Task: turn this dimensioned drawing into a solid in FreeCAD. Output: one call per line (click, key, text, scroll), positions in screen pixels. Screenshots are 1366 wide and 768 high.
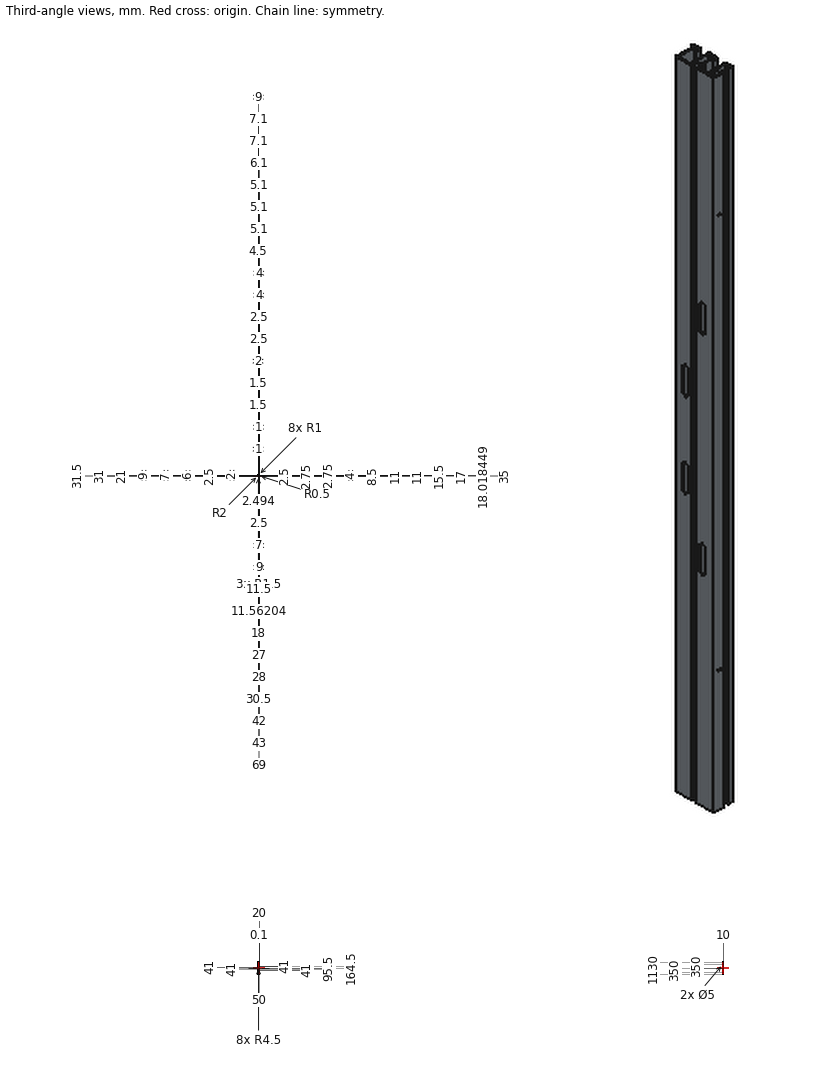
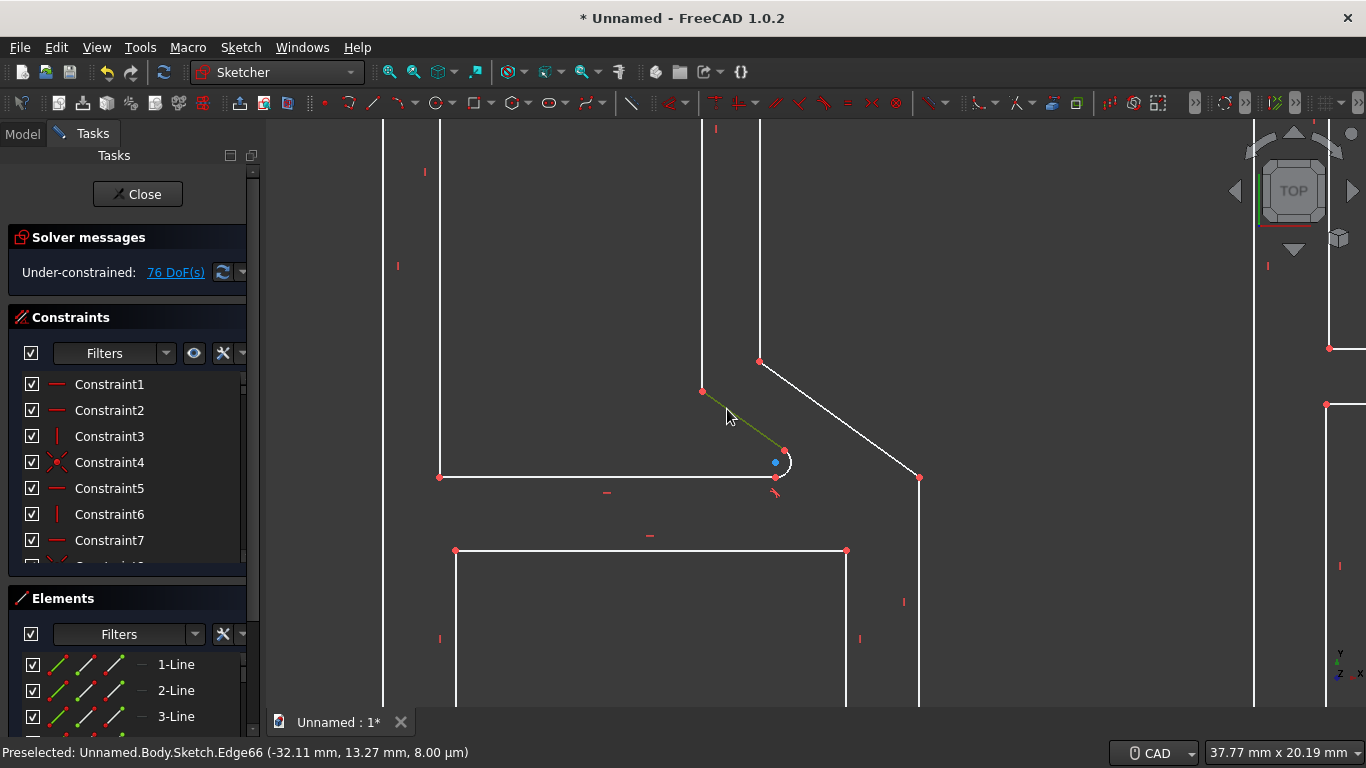
scroll(786, 473, up, 2)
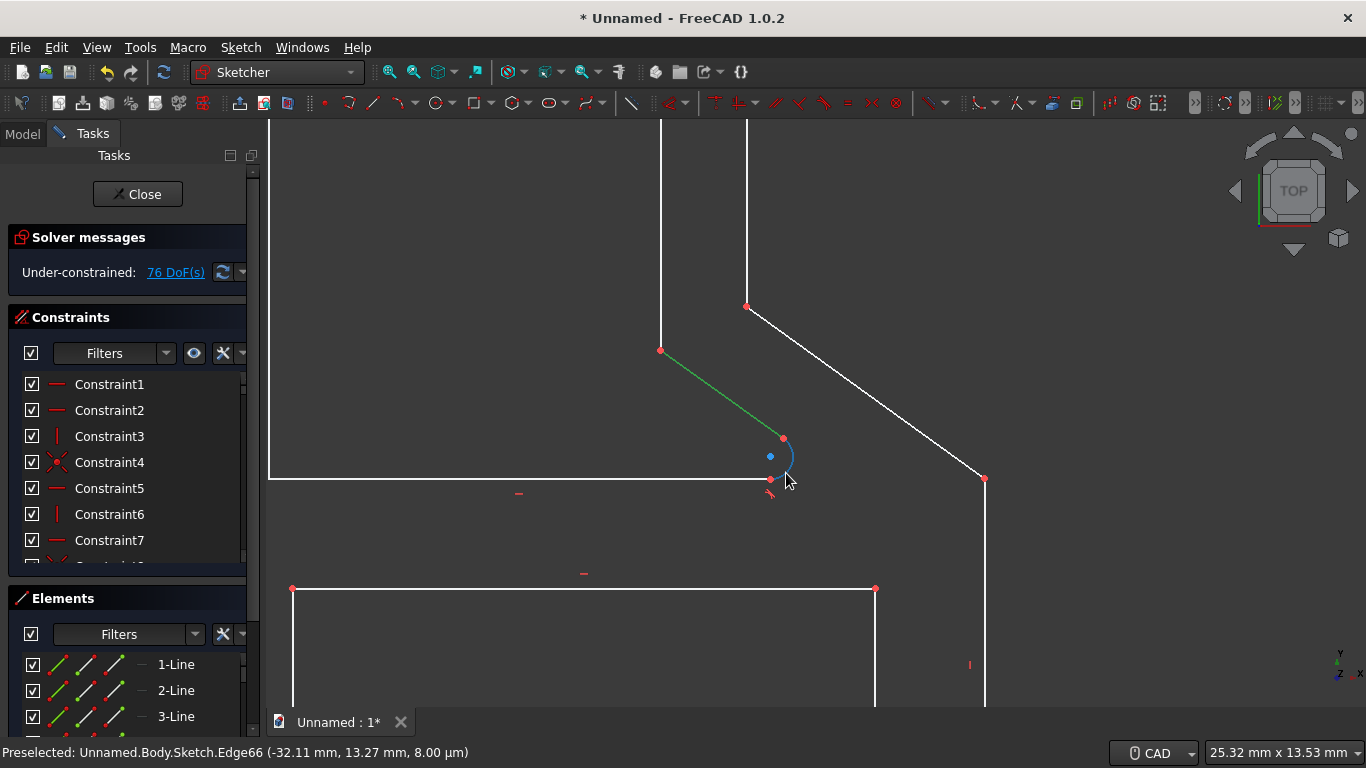
click(786, 473)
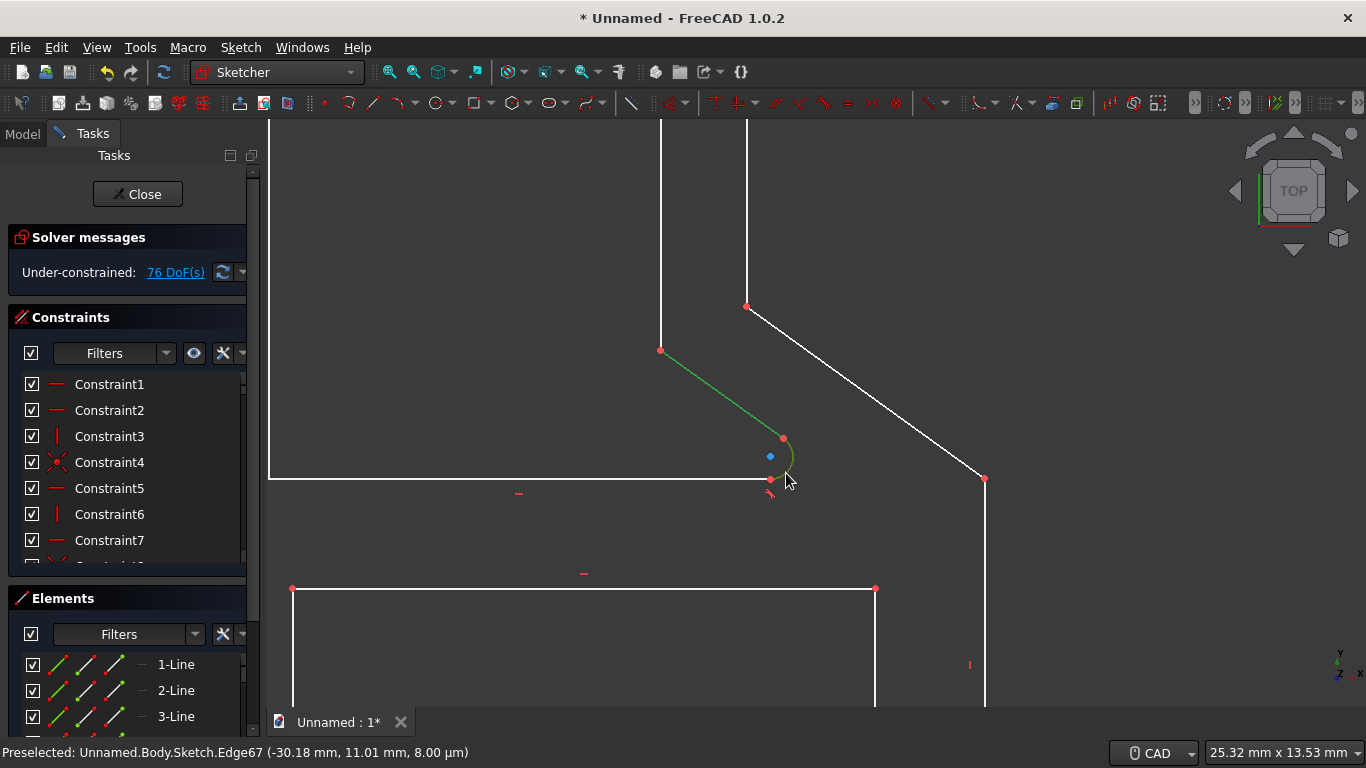
key(t)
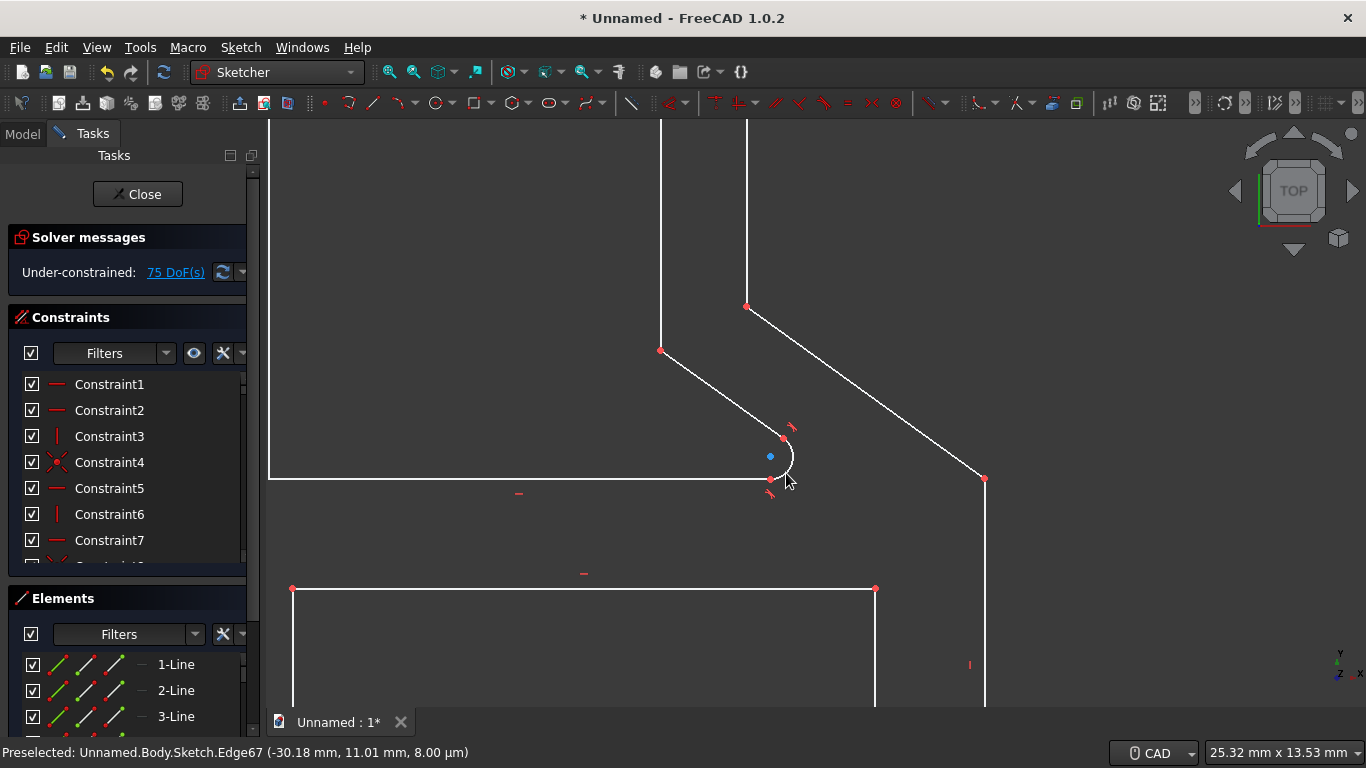
scroll(792, 468, down, 8)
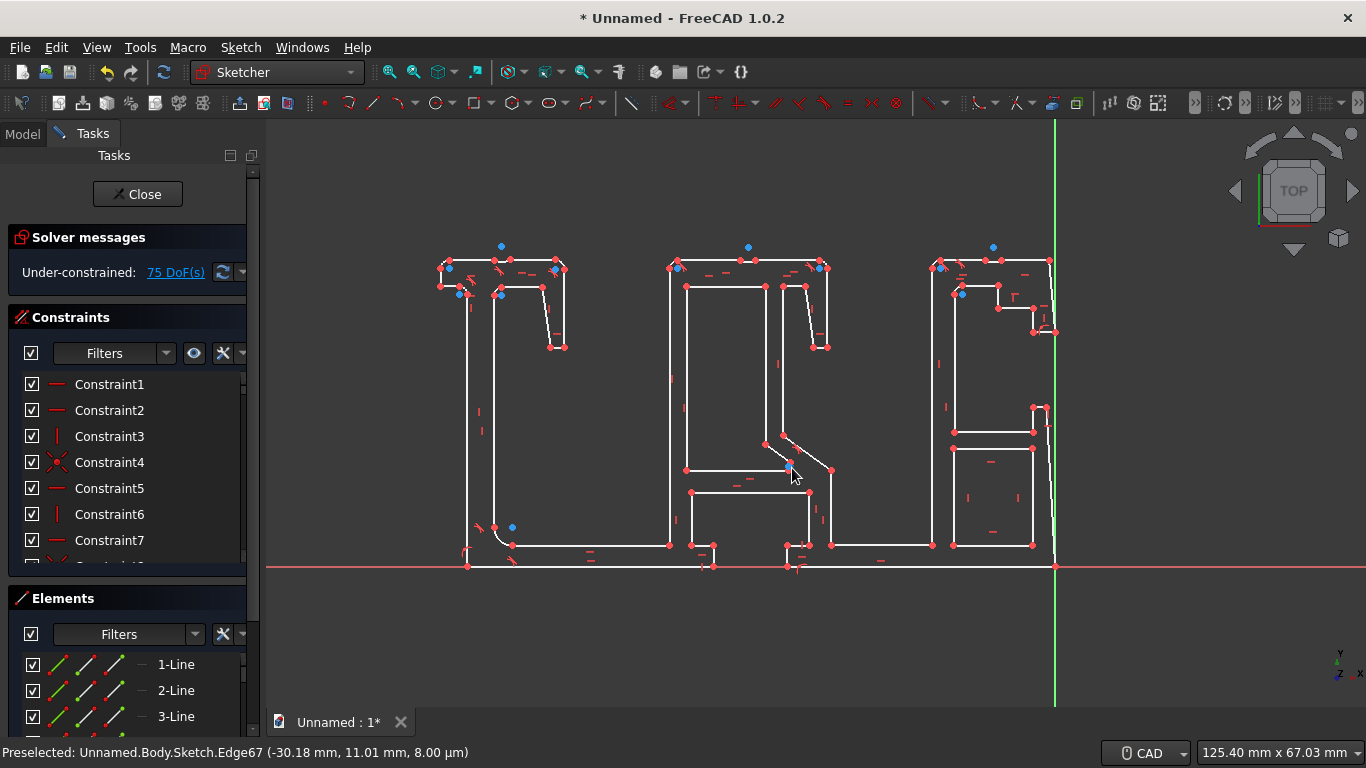
scroll(1053, 519, up, 9)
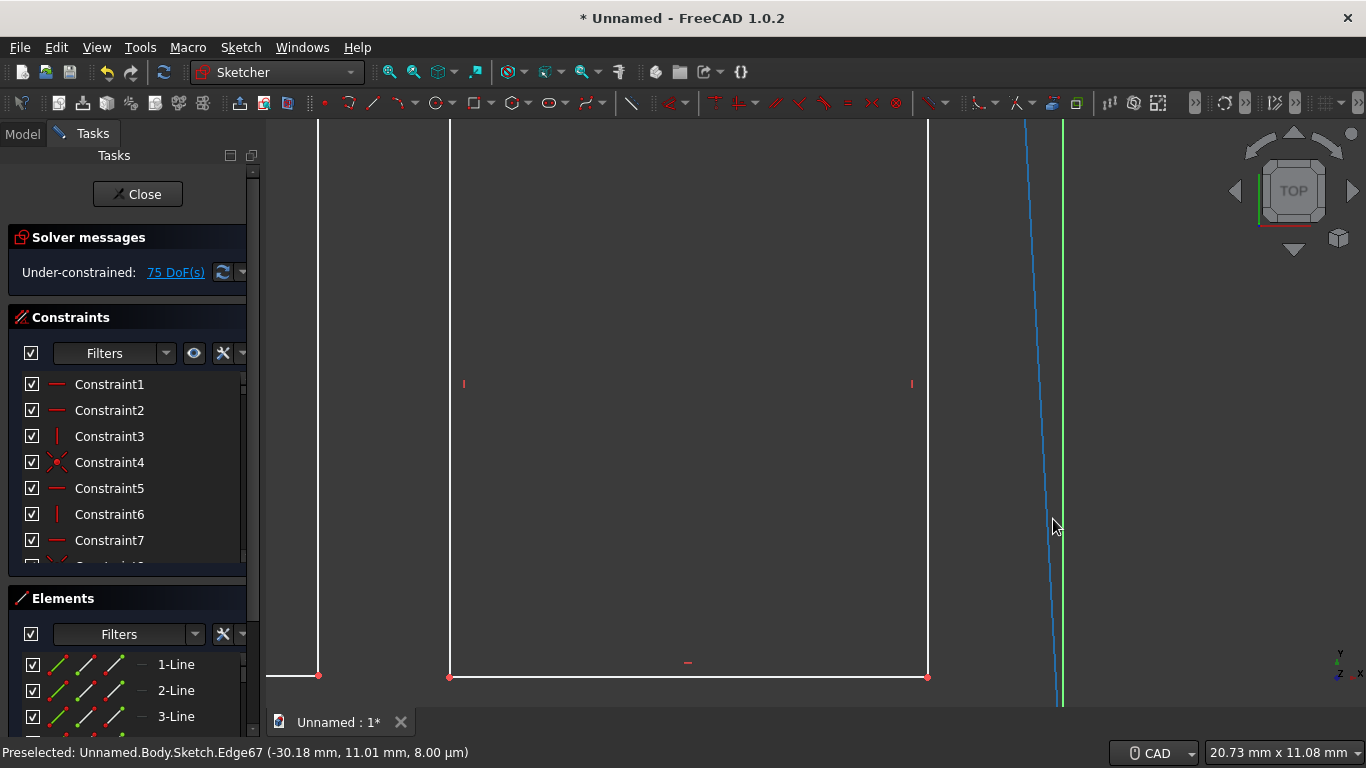
click(1047, 514)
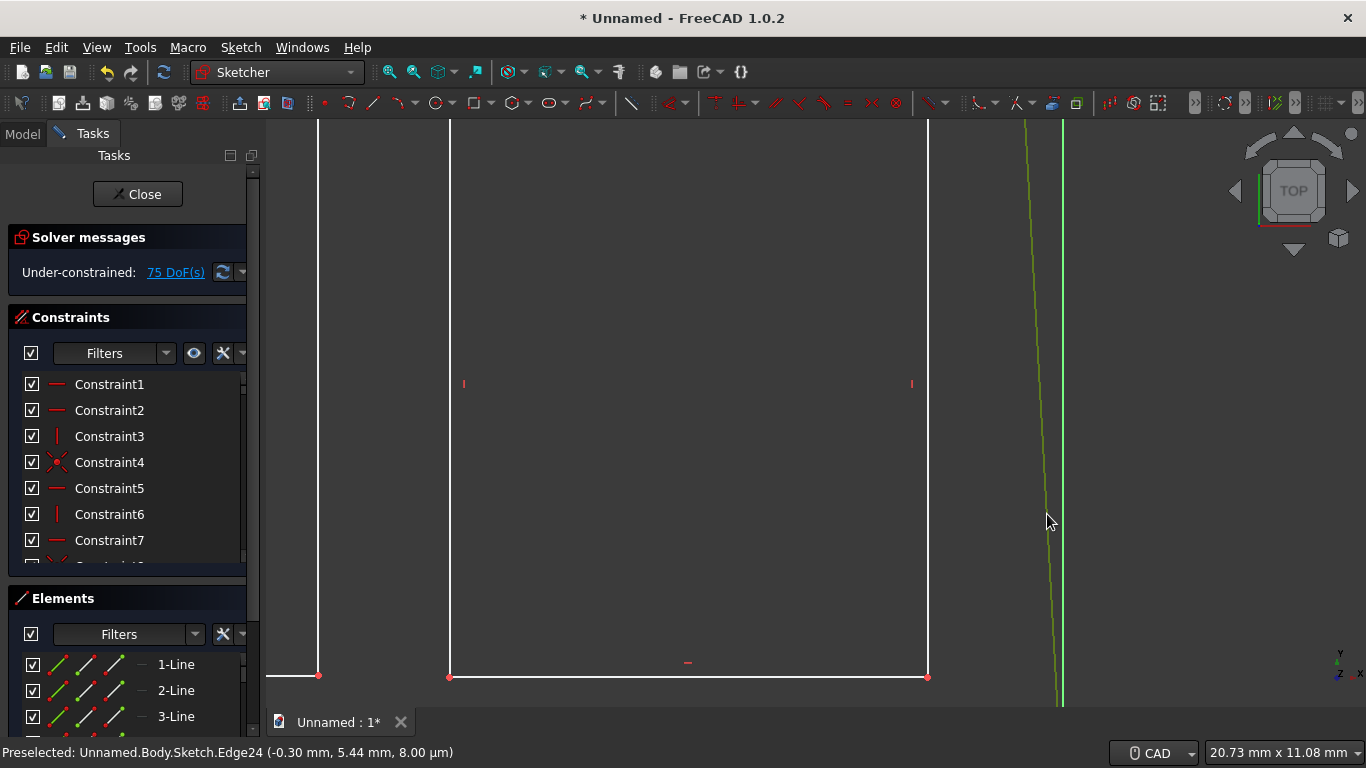
key(v)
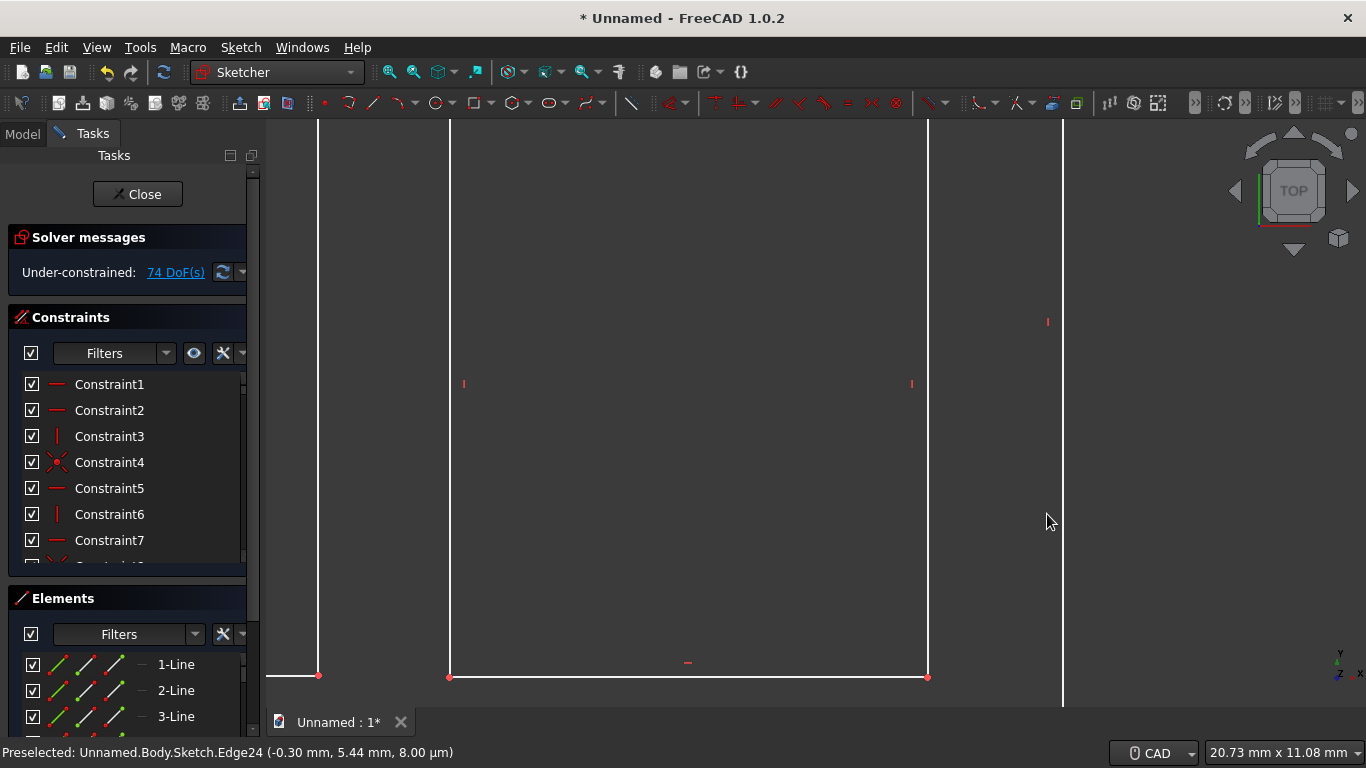
scroll(1053, 520, down, 9)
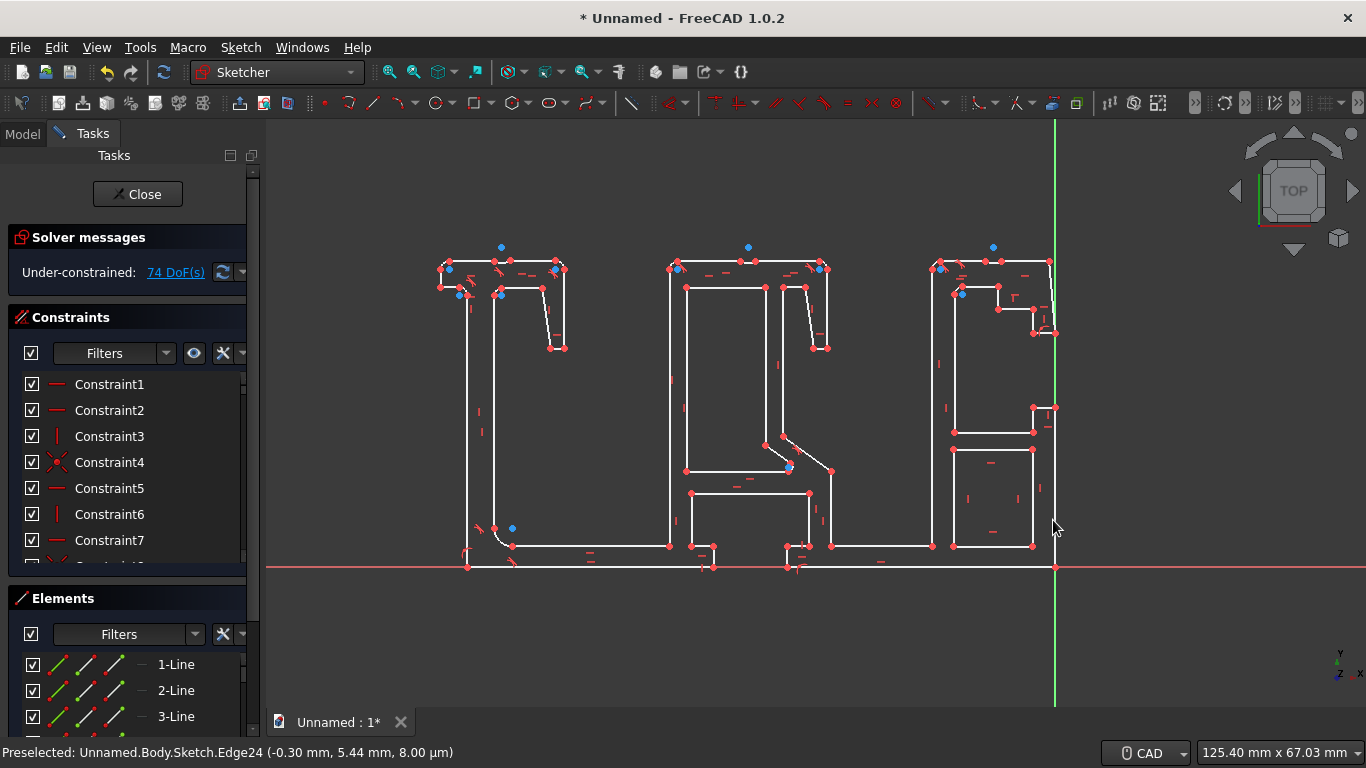
scroll(1053, 312, up, 11)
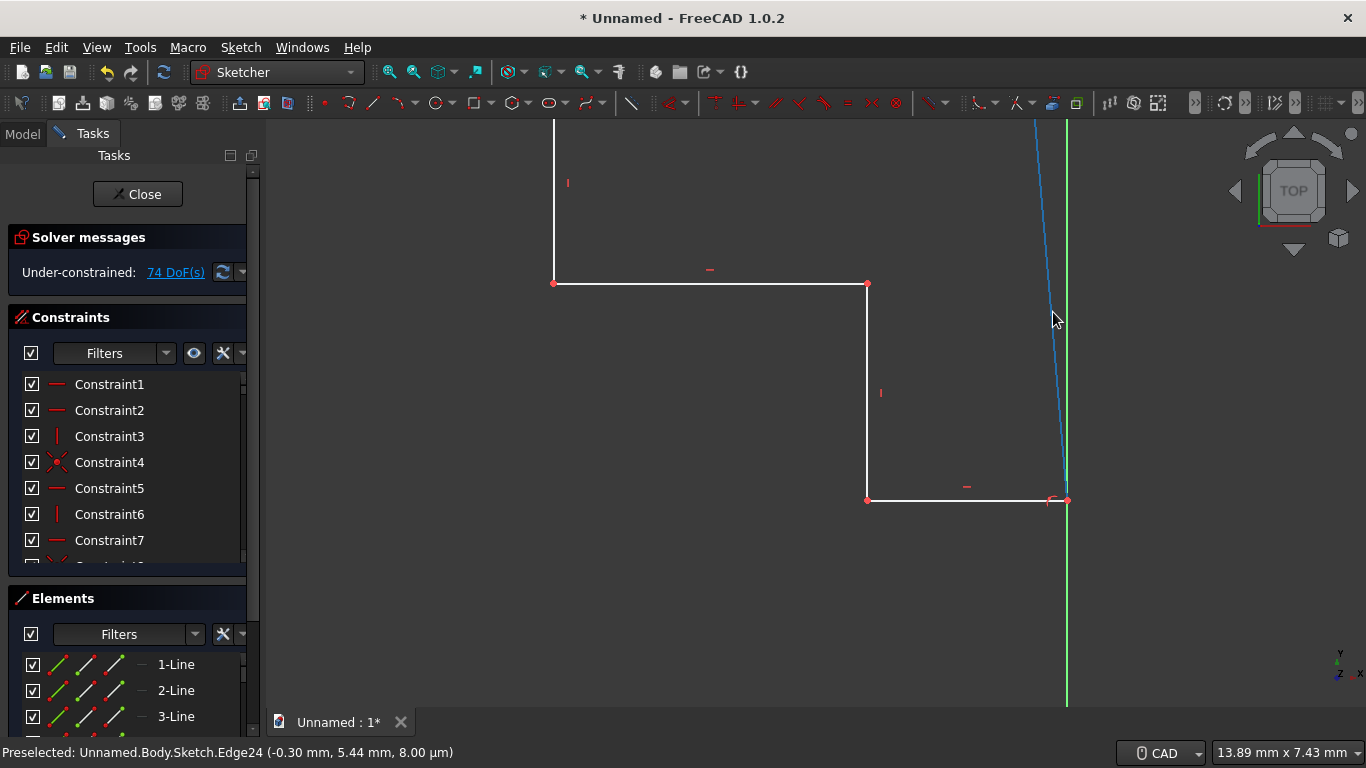
click(1051, 305)